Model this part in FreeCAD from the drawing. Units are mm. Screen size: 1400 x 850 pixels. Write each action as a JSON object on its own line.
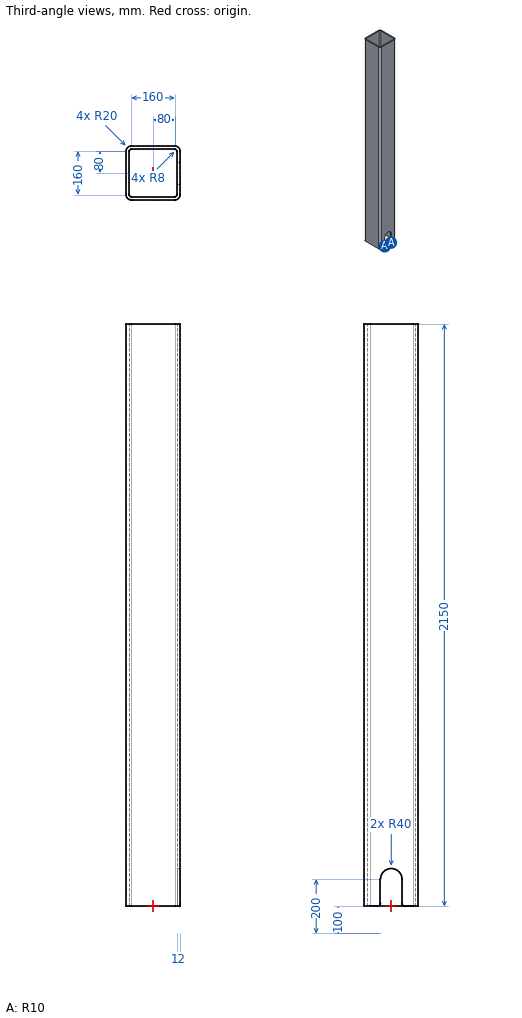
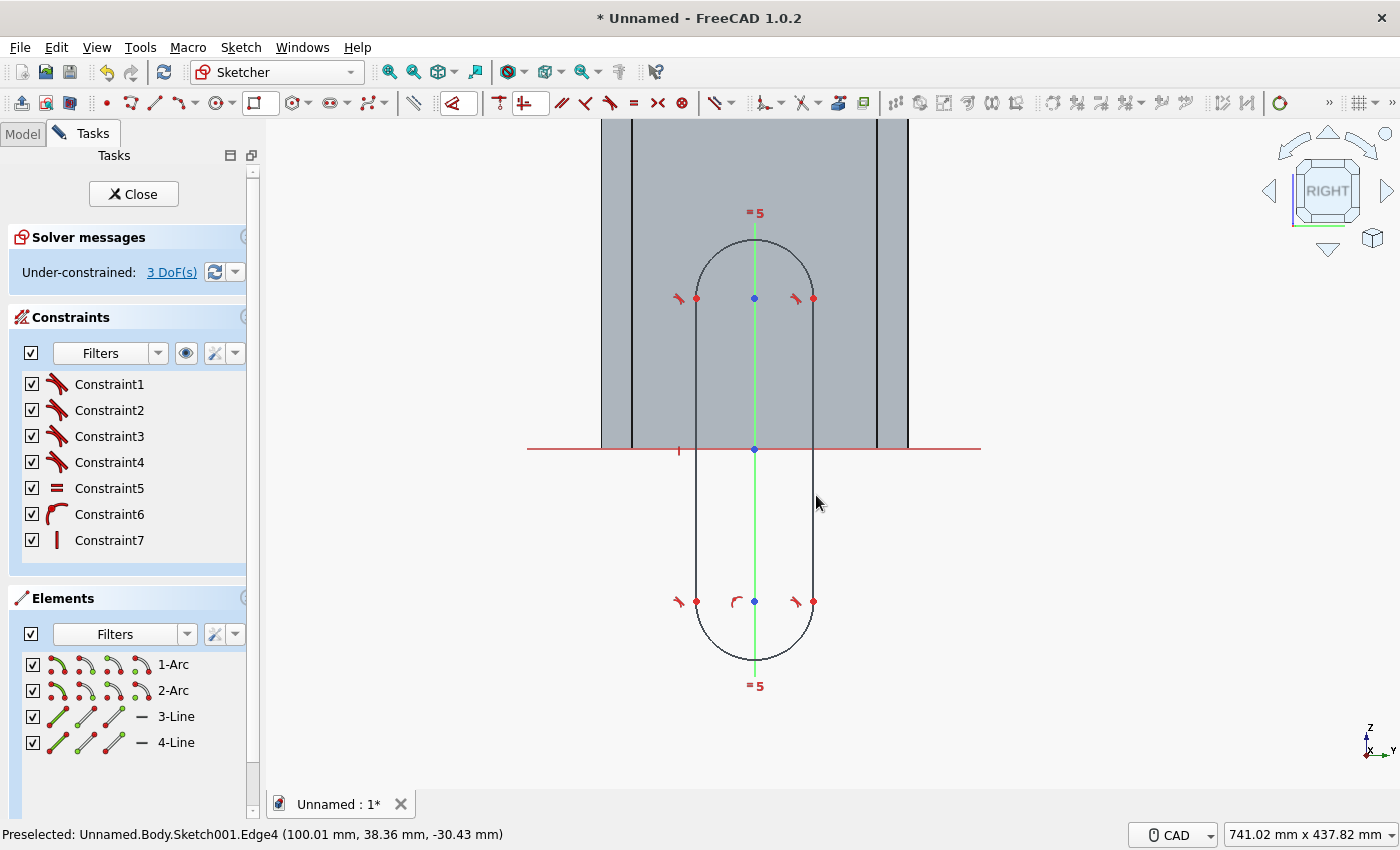
{"action": "left_click", "coordinate": [720, 649]}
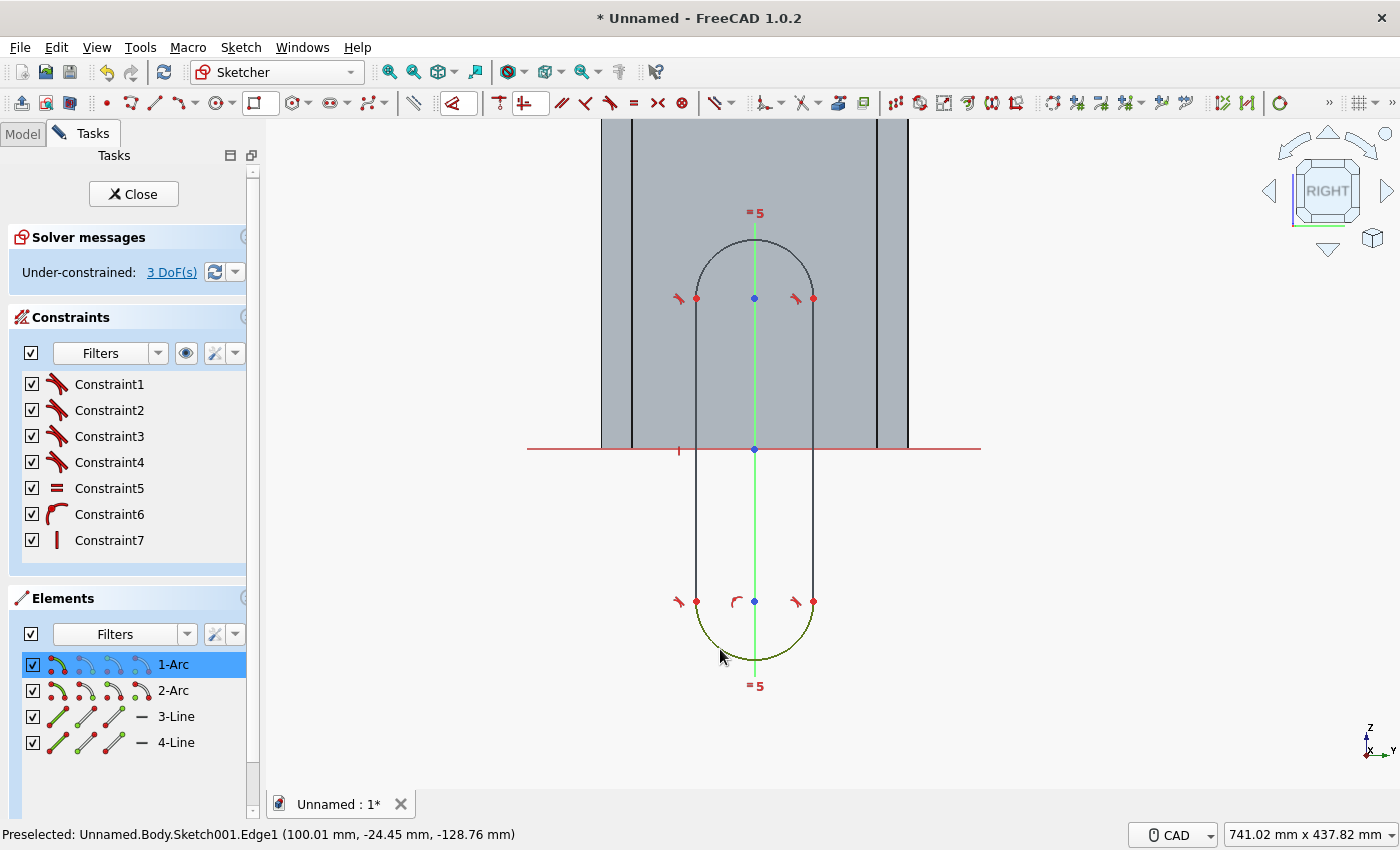
{"action": "key", "text": "k r"}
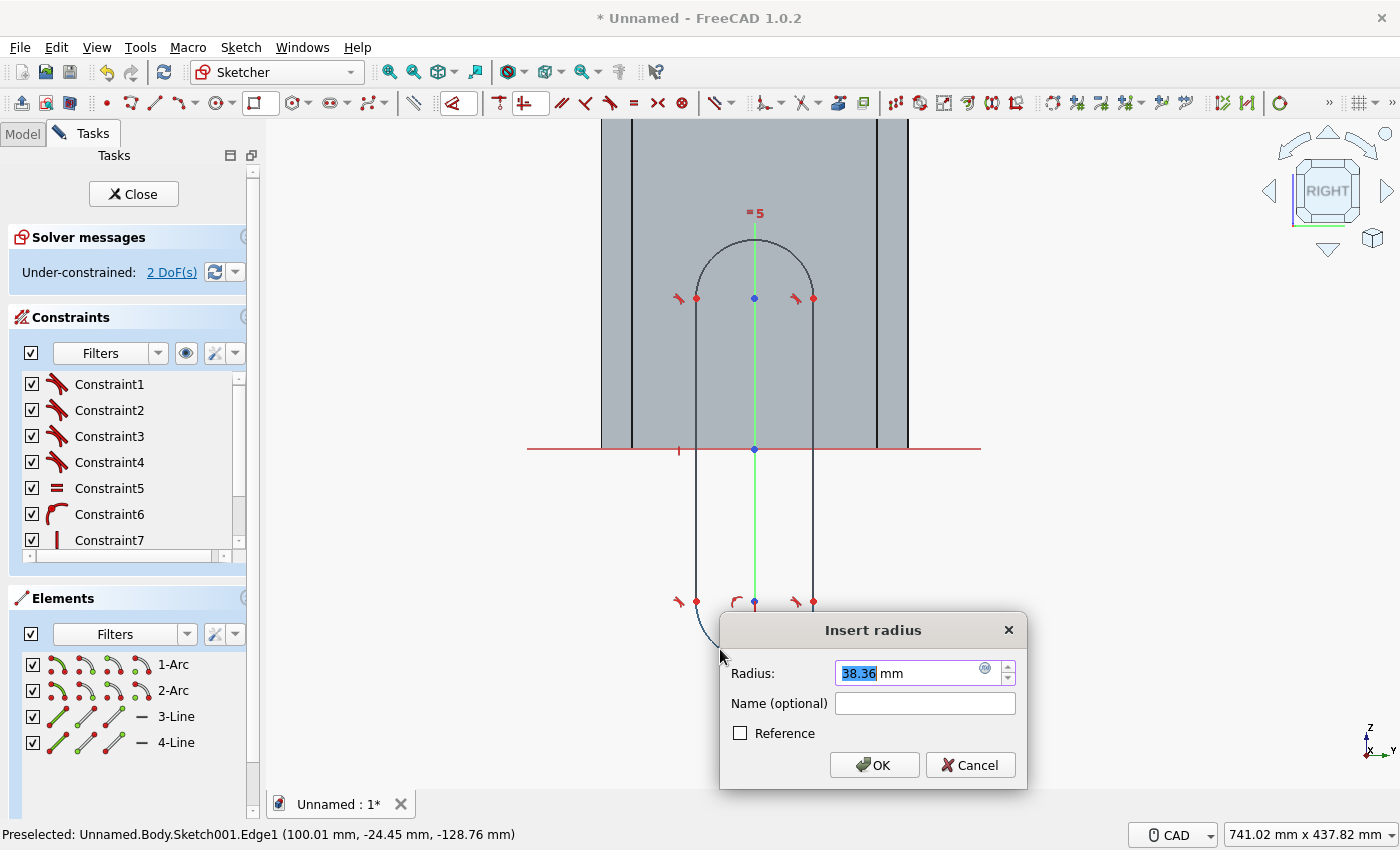
{"action": "type", "text": "40"}
{"action": "key", "text": "Return"}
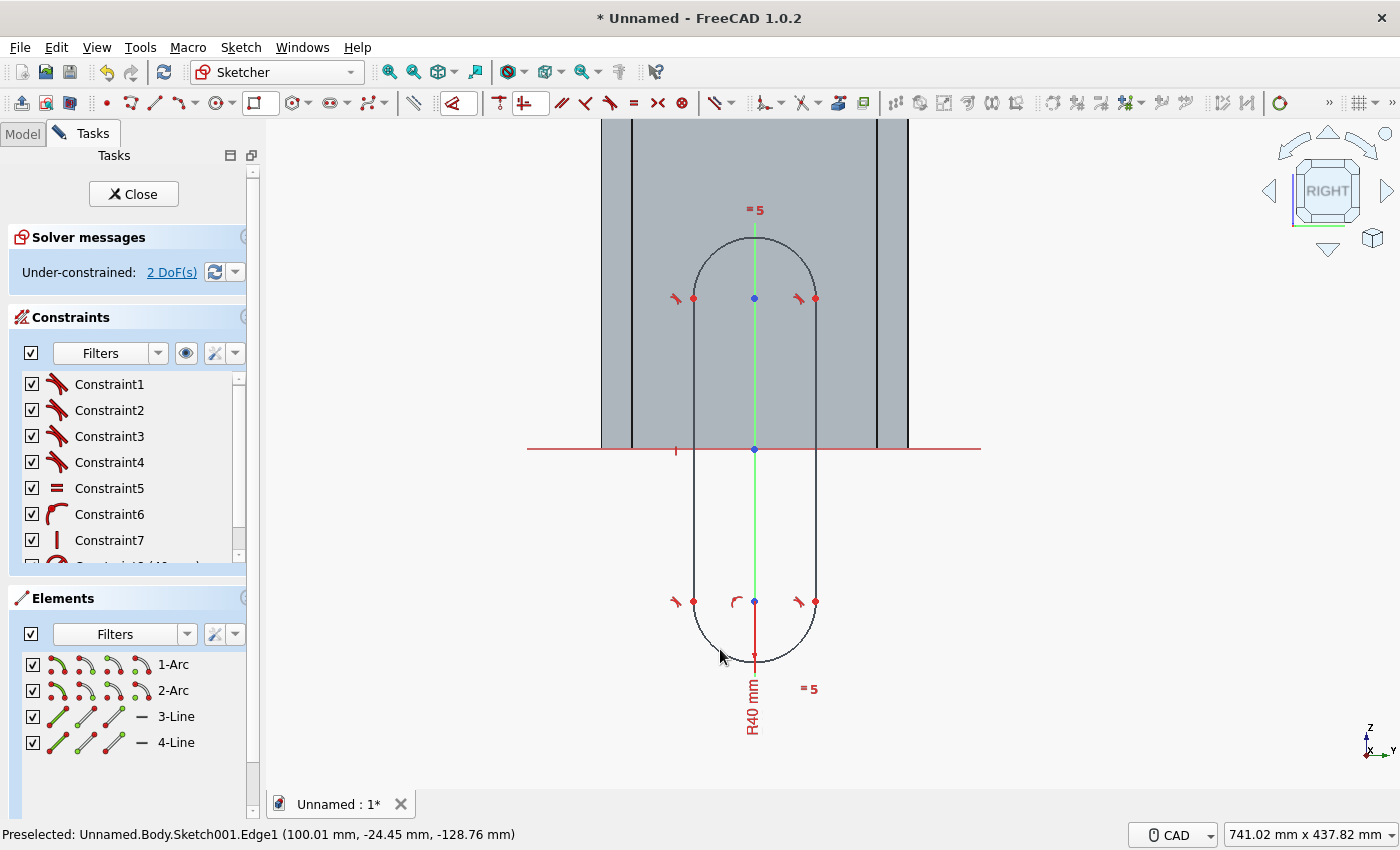
{"action": "left_click", "coordinate": [694, 510]}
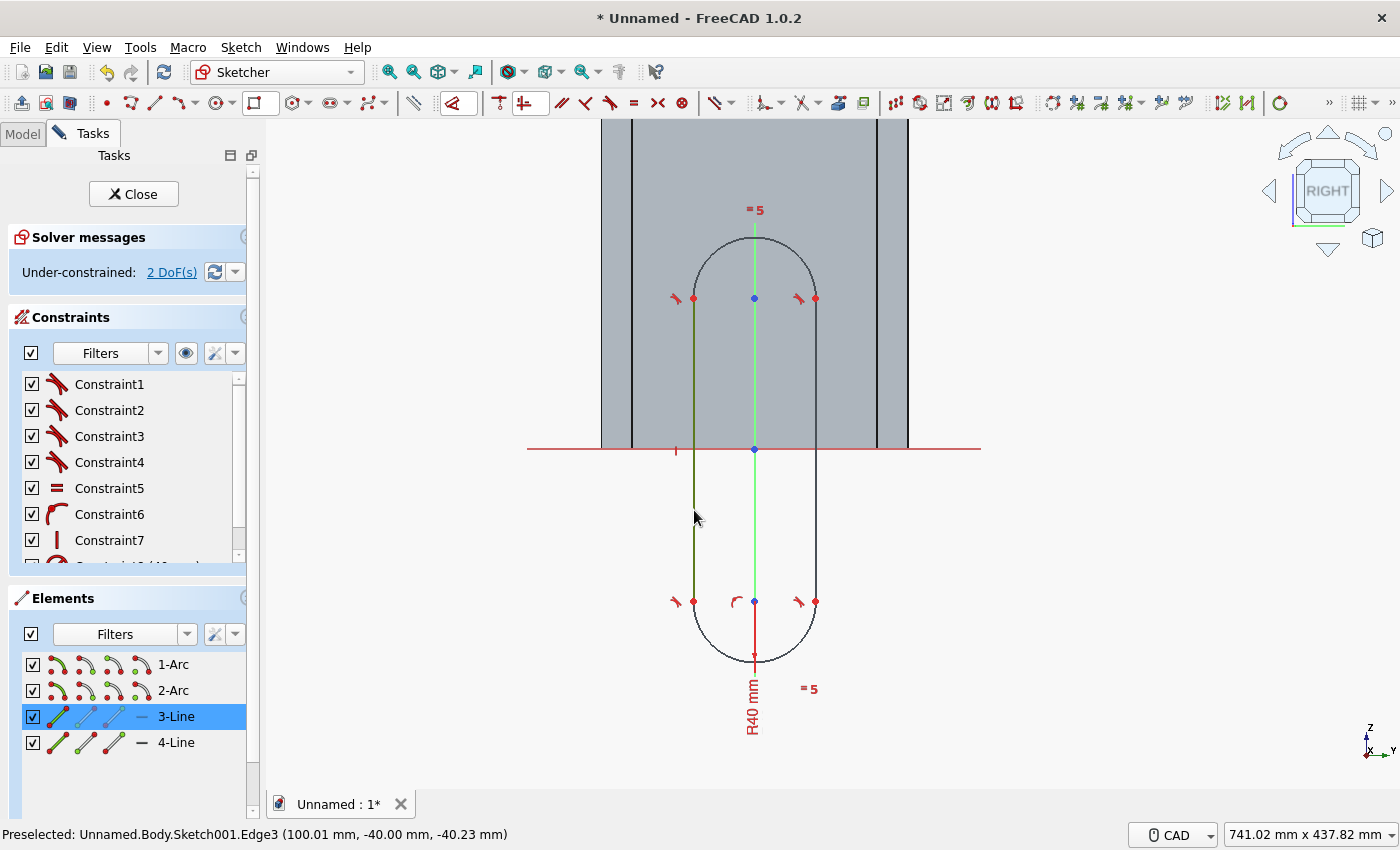
{"action": "key", "text": "i"}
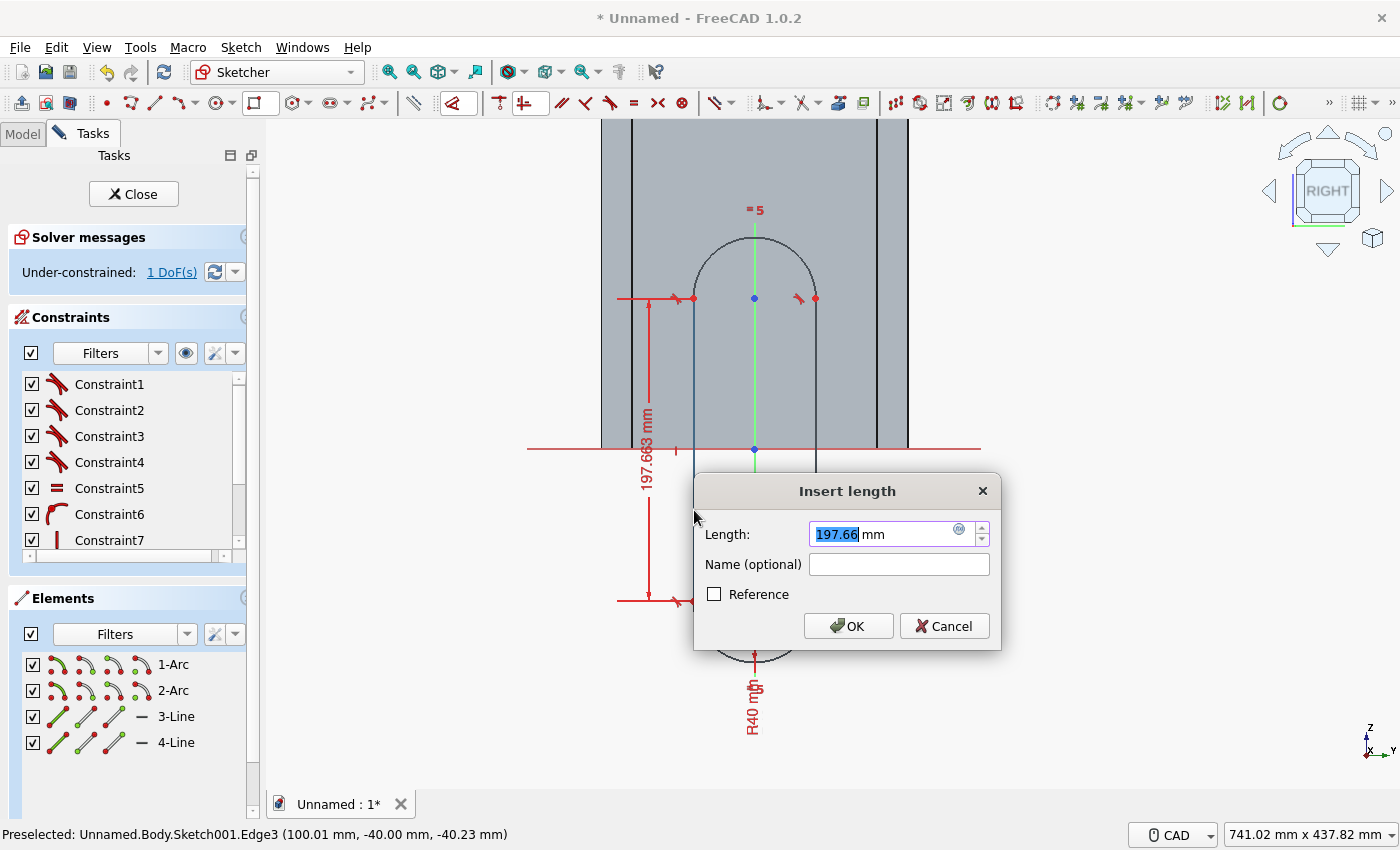
{"action": "type", "text": "200"}
{"action": "key", "text": "Return"}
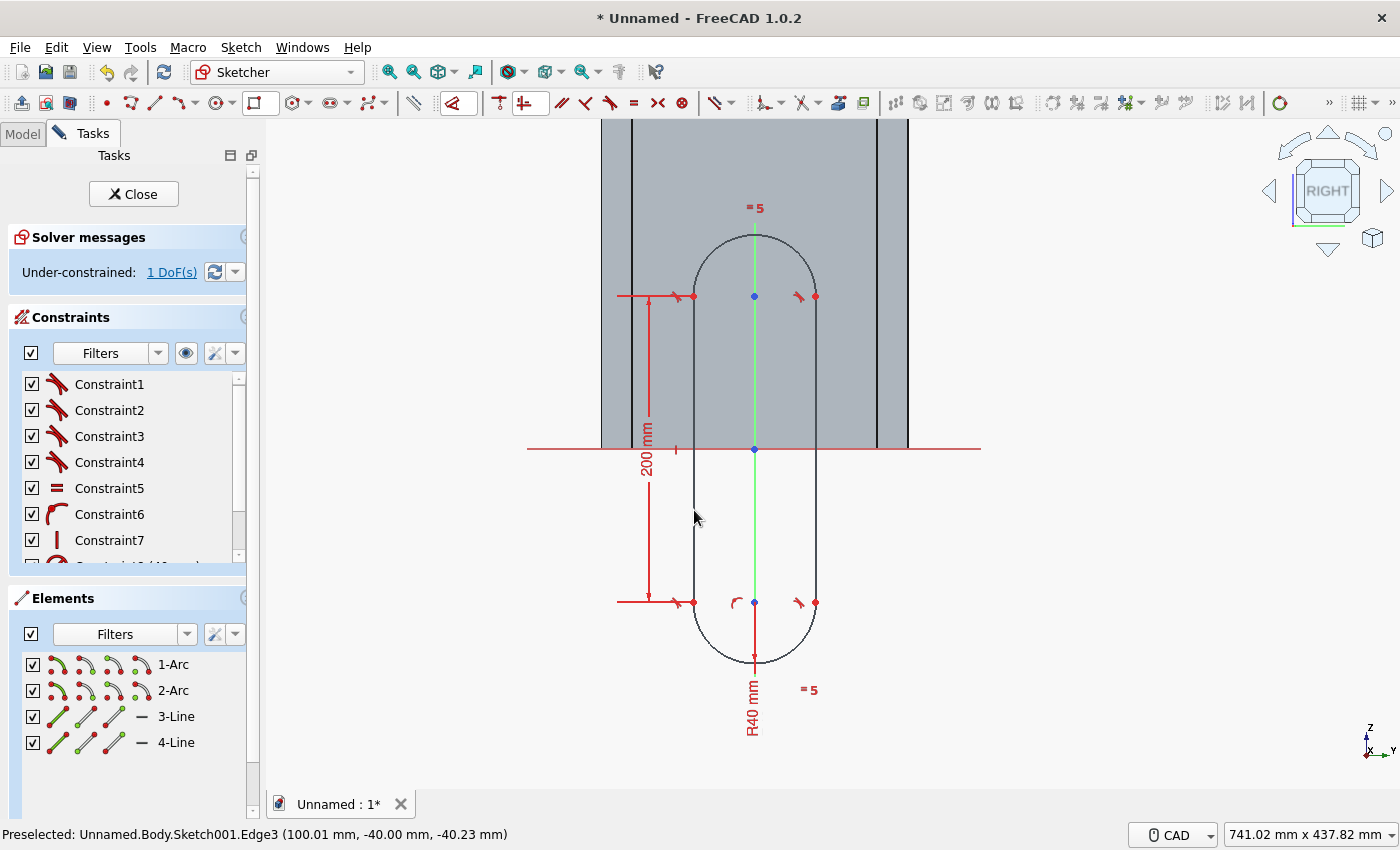
{"action": "left_click", "coordinate": [694, 602]}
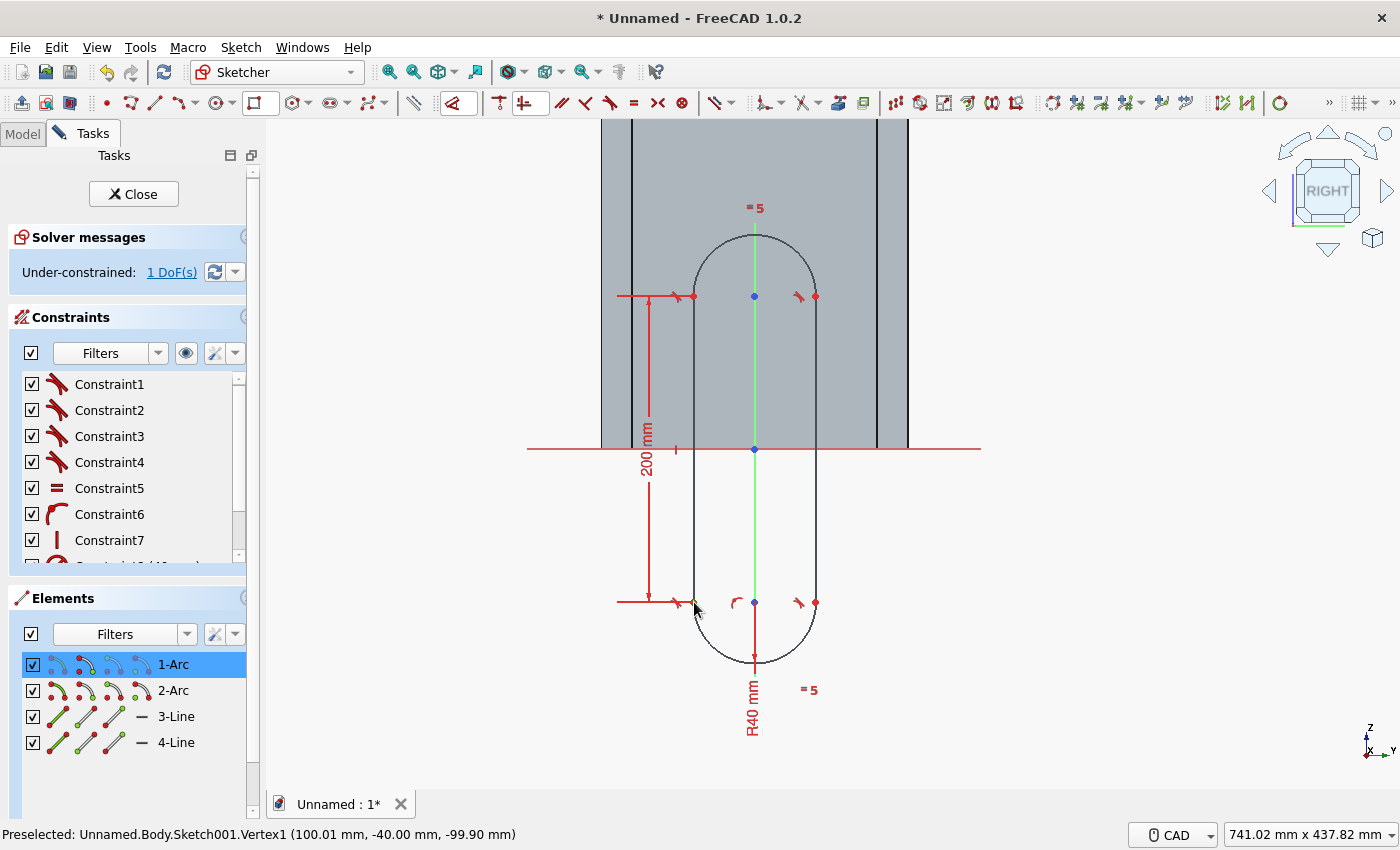
{"action": "left_click", "coordinate": [472, 104]}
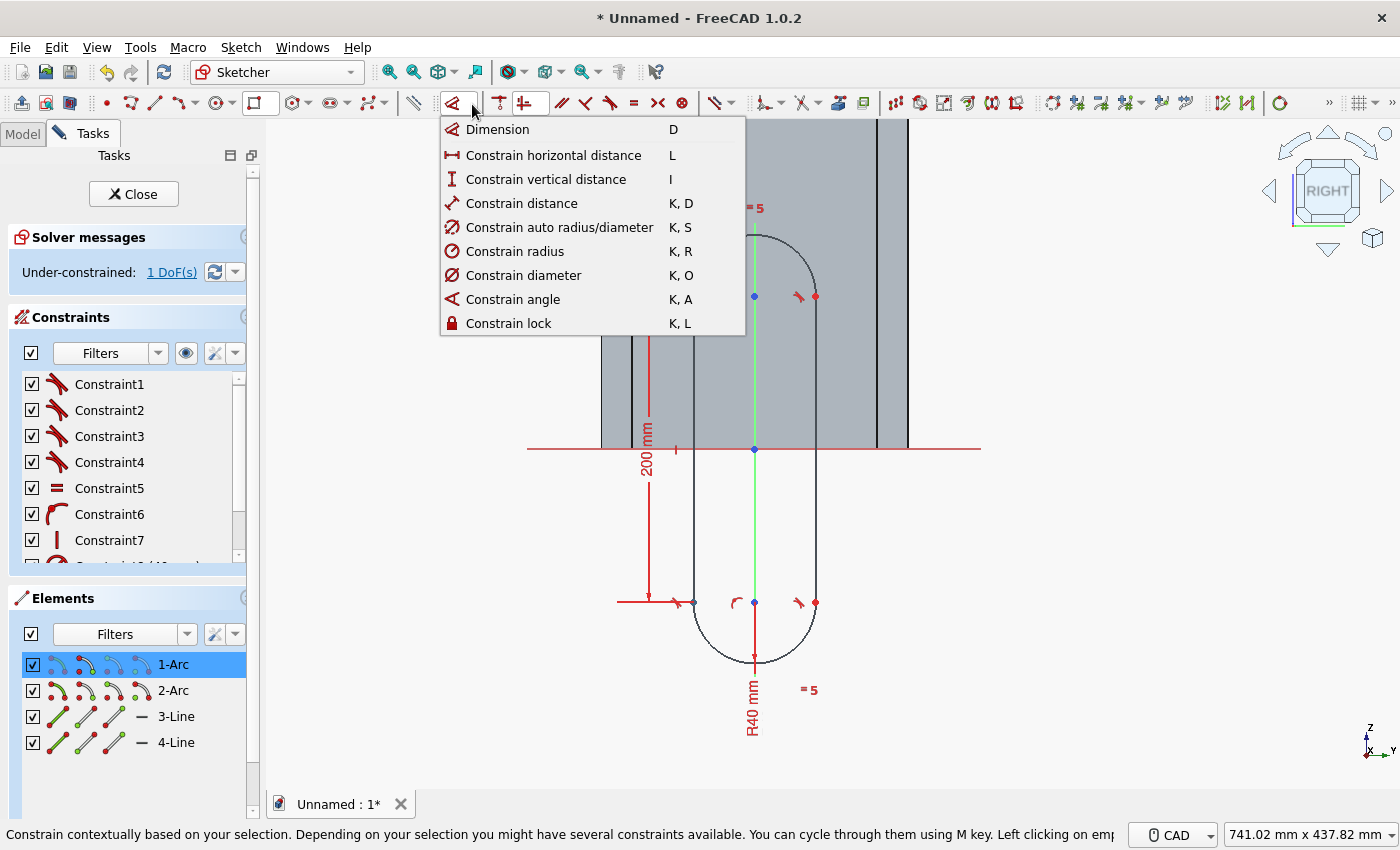
{"action": "left_click", "coordinate": [593, 179]}